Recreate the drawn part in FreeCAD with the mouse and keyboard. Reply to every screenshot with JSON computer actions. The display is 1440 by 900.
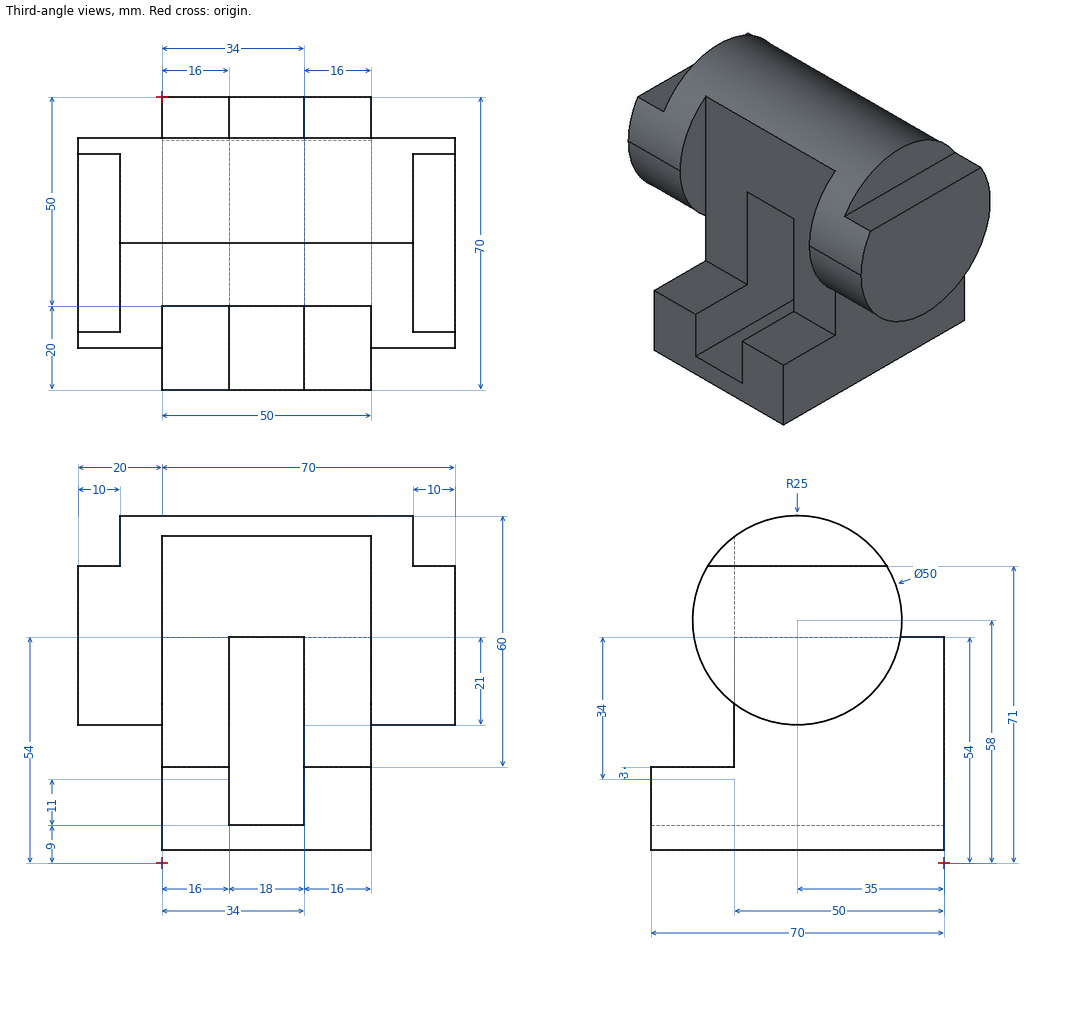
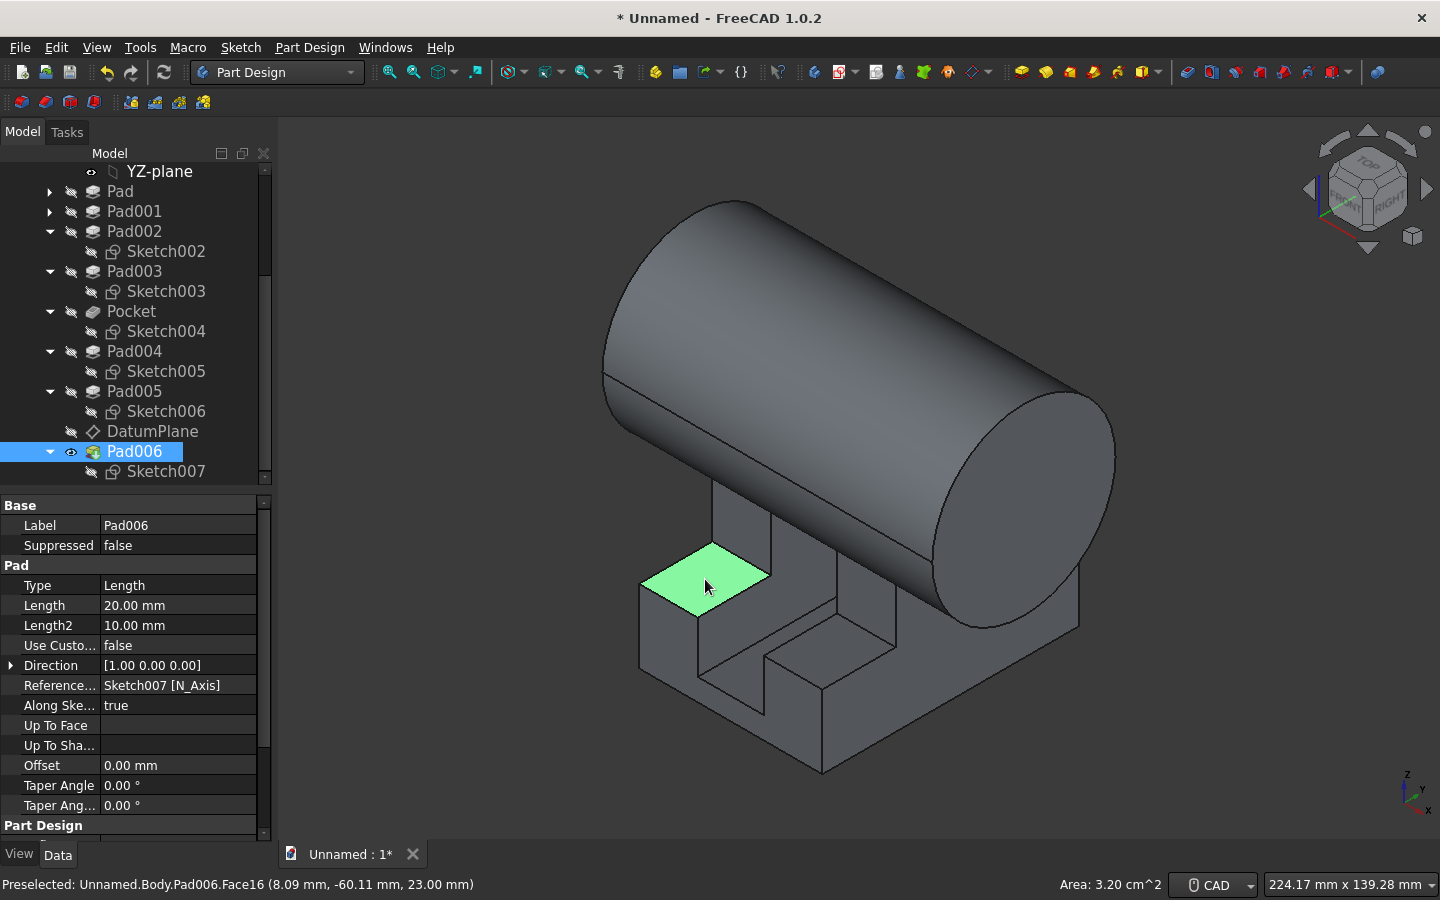
{"action": "left_click", "coordinate": [840, 72]}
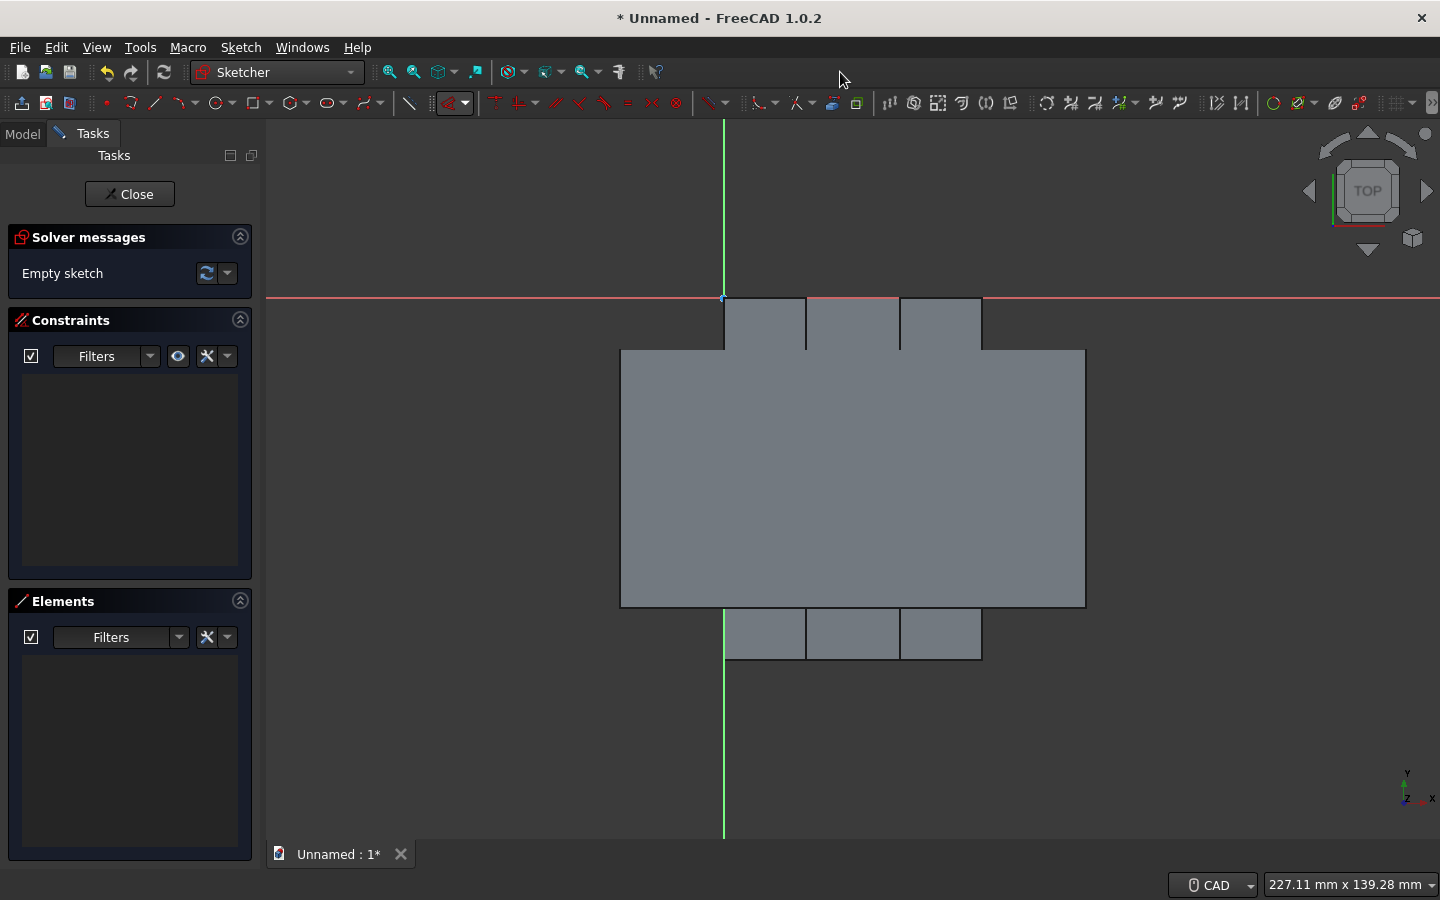
{"action": "key", "text": "q s"}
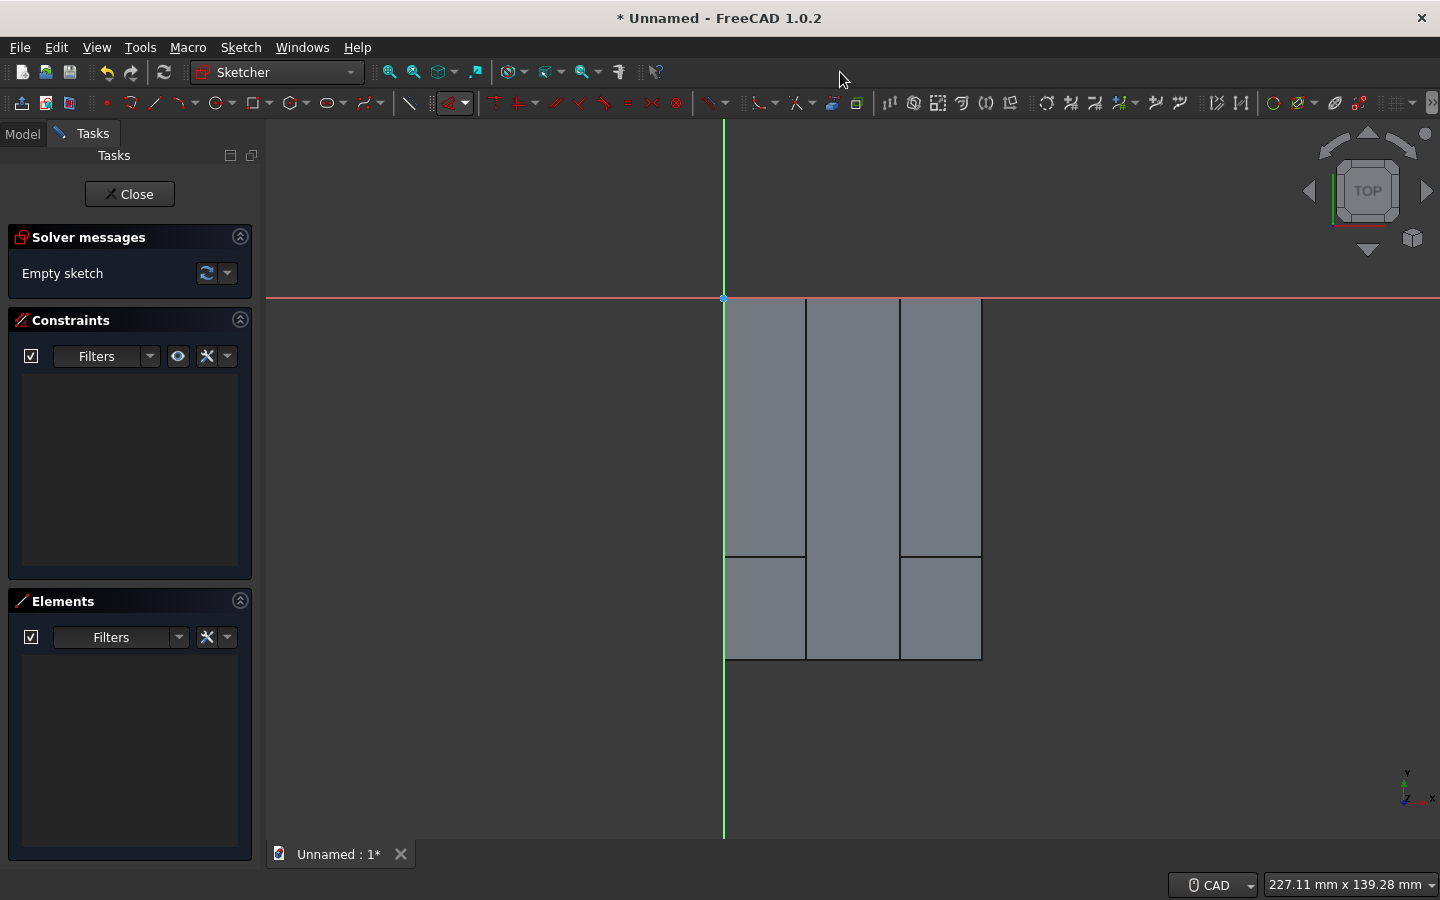
{"action": "key", "text": "g r"}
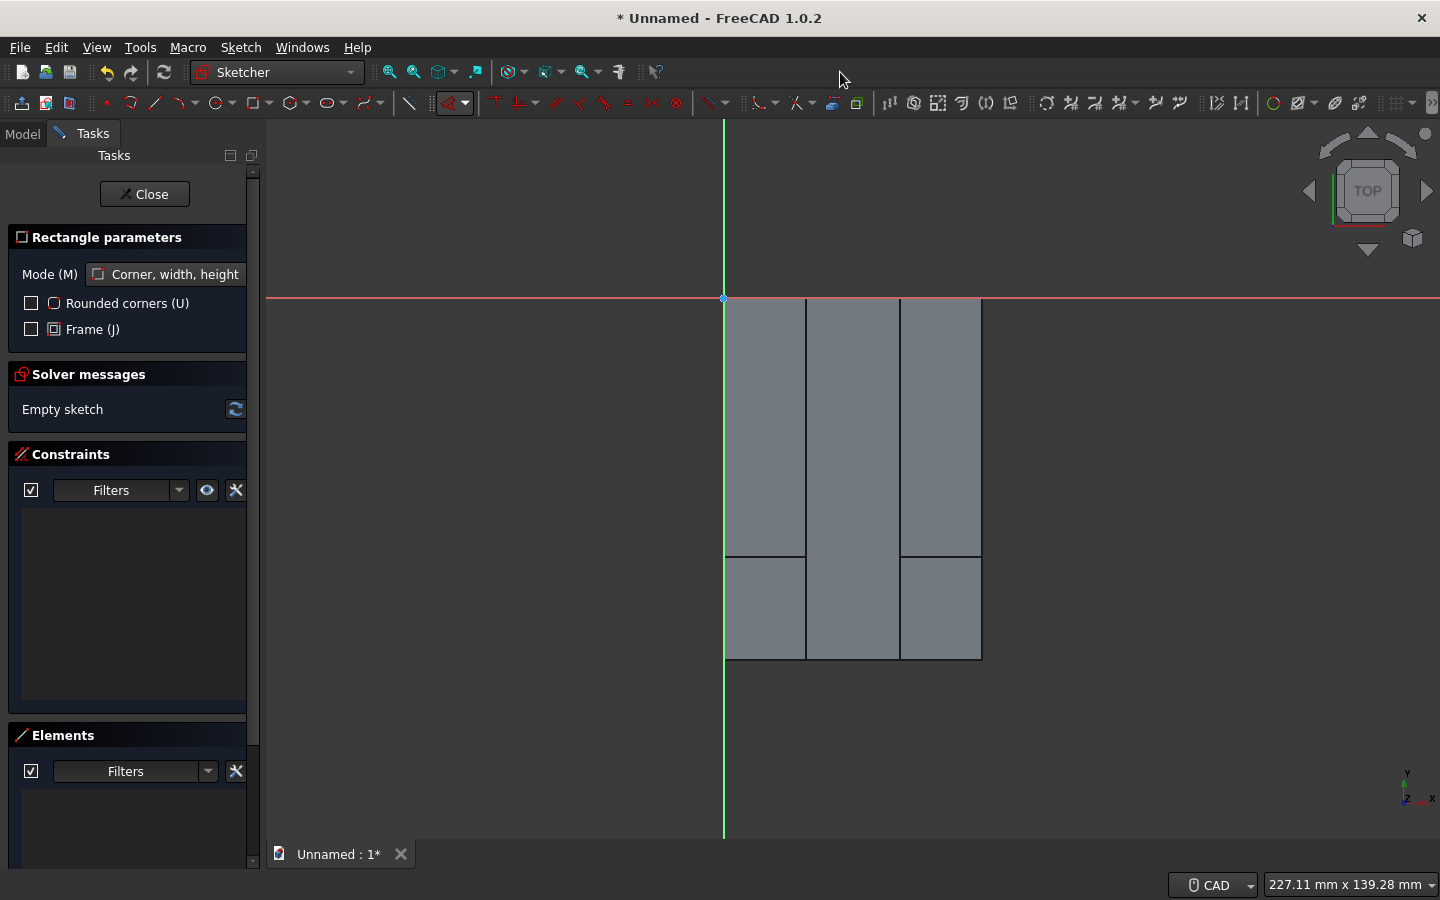
{"action": "left_click", "coordinate": [724, 557]}
{"action": "mouse_move", "coordinate": [982, 660]}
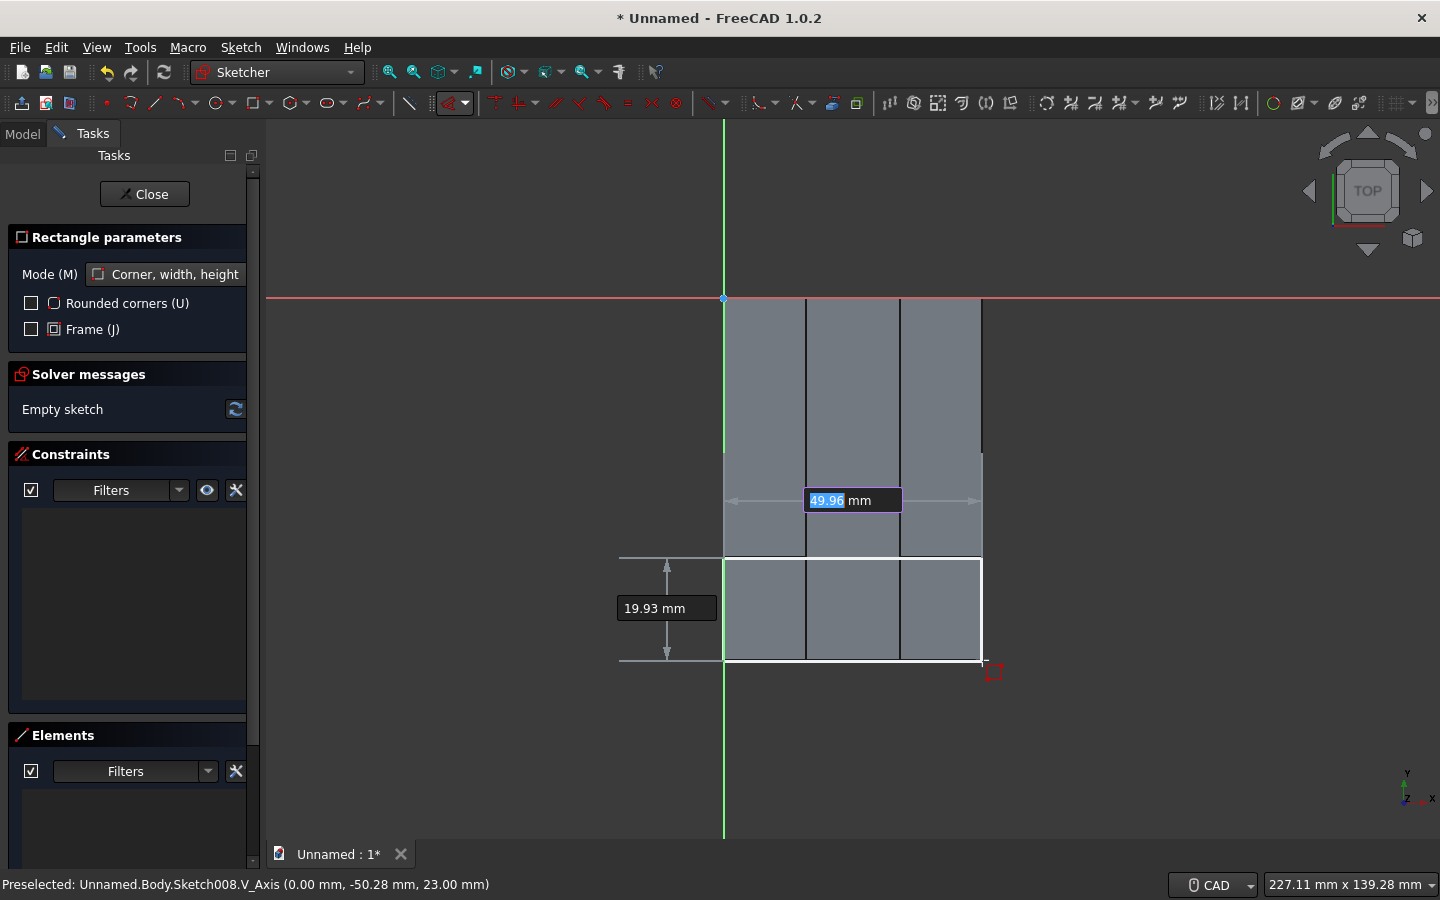
{"action": "type", "text": "50"}
{"action": "key", "text": "Tab"}
{"action": "type", "text": "20"}
{"action": "key", "text": "Return"}
{"action": "key", "text": "Escape"}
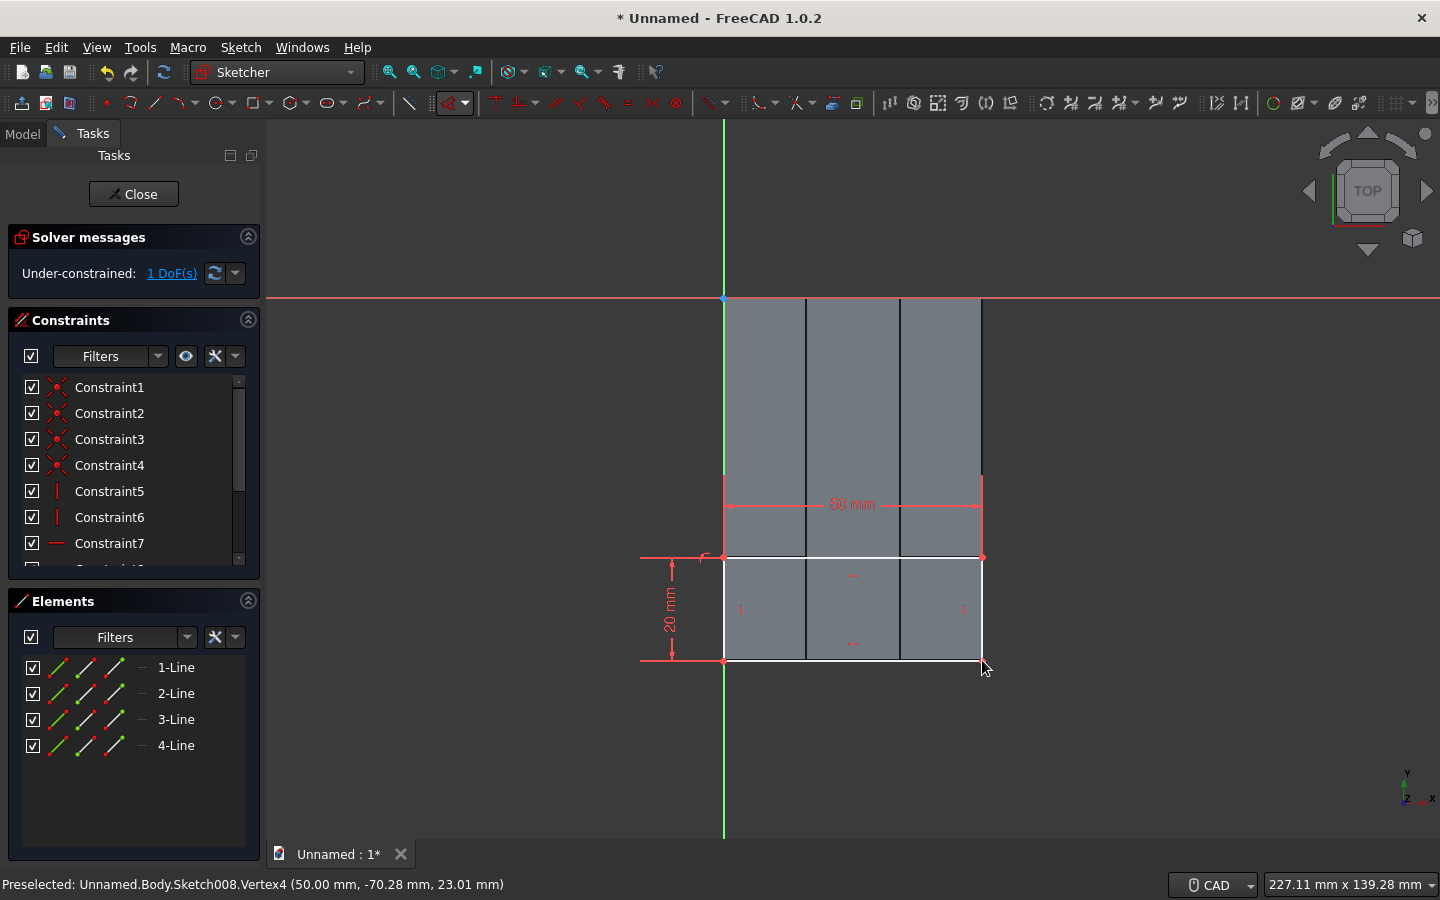
{"action": "left_click", "coordinate": [724, 558]}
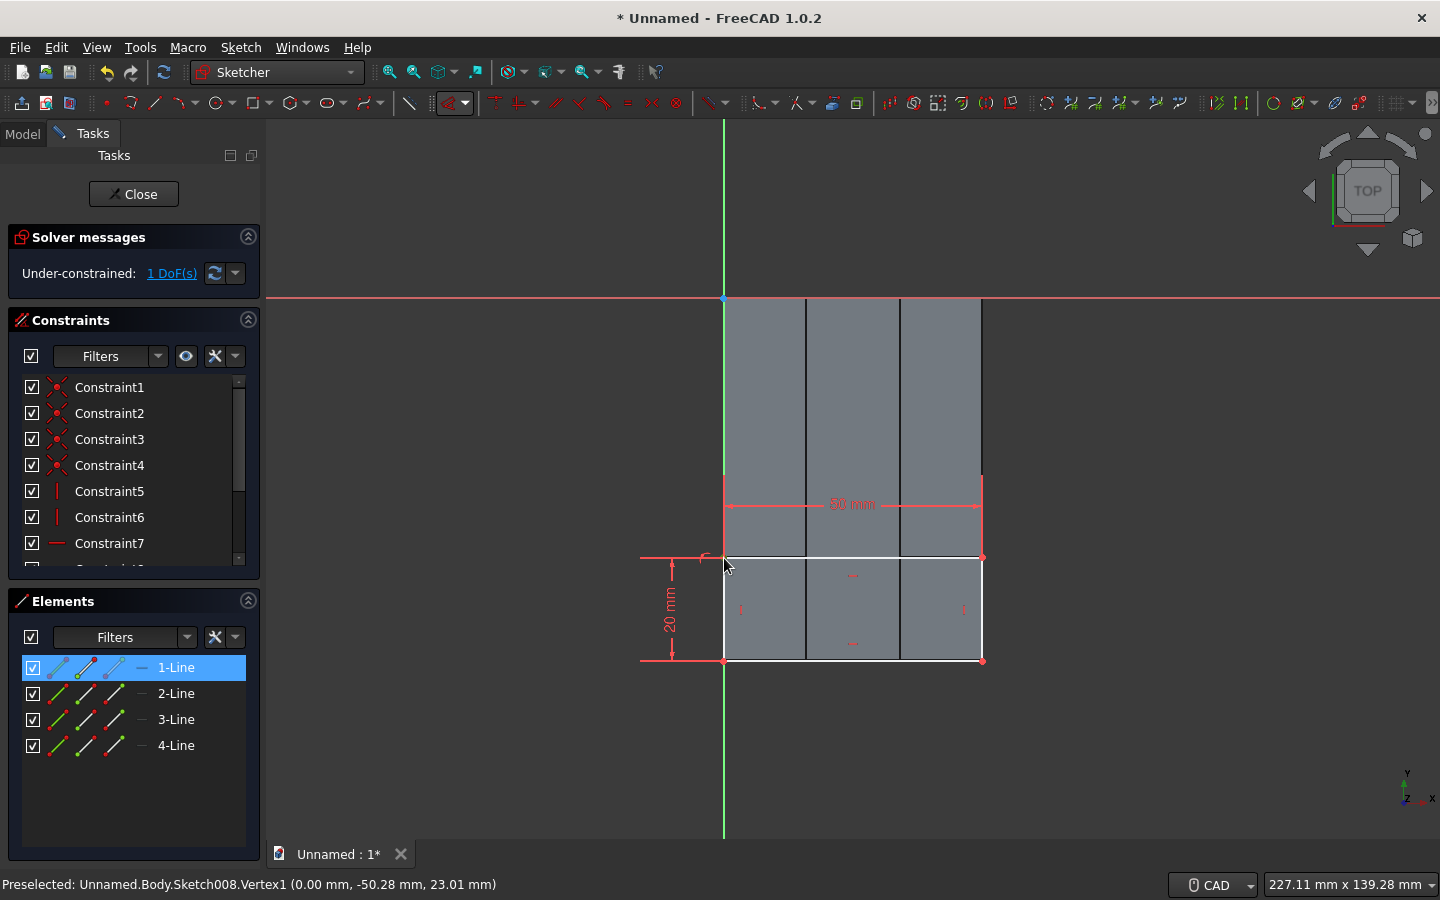
{"action": "key", "text": "i"}